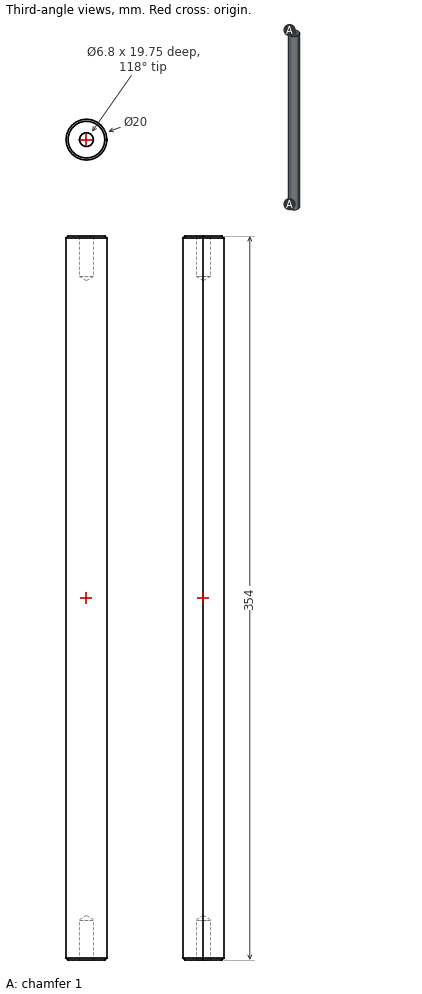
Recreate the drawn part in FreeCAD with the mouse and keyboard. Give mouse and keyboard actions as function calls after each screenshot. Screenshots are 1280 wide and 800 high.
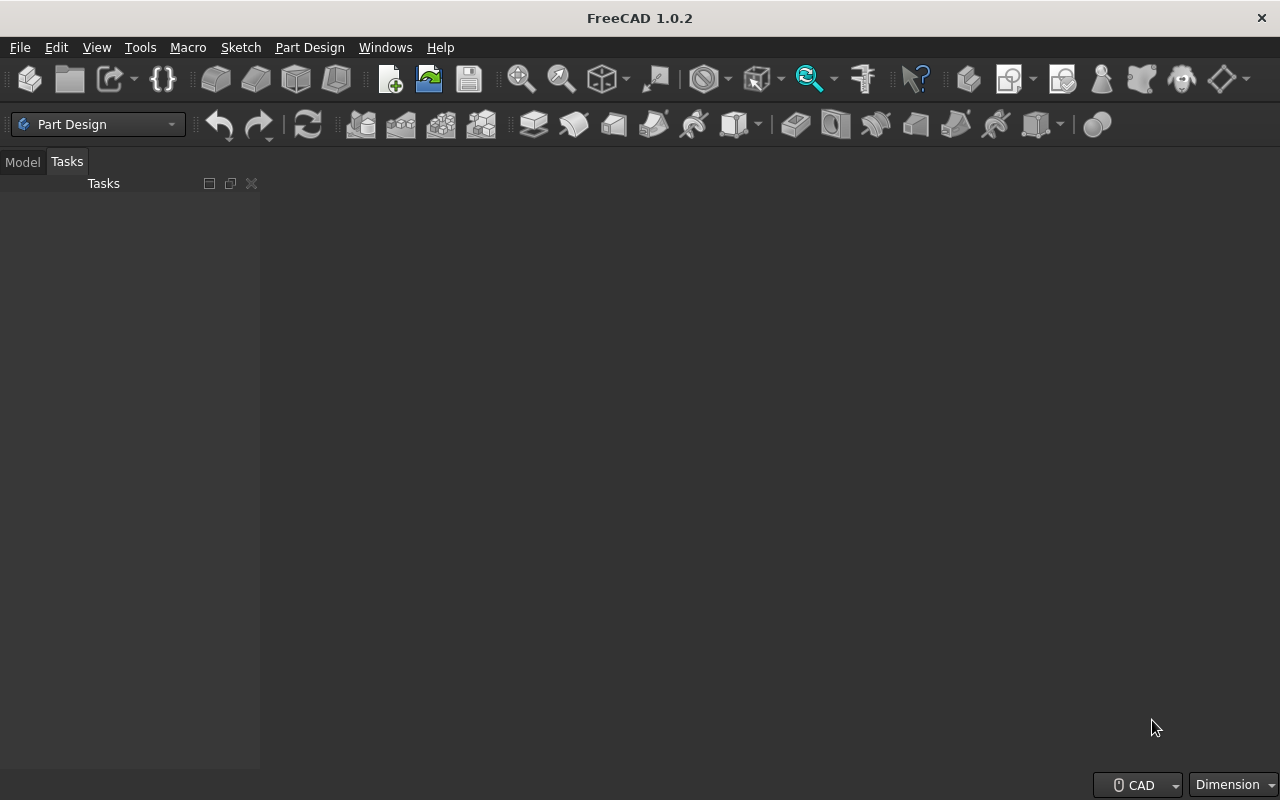
click(390, 80)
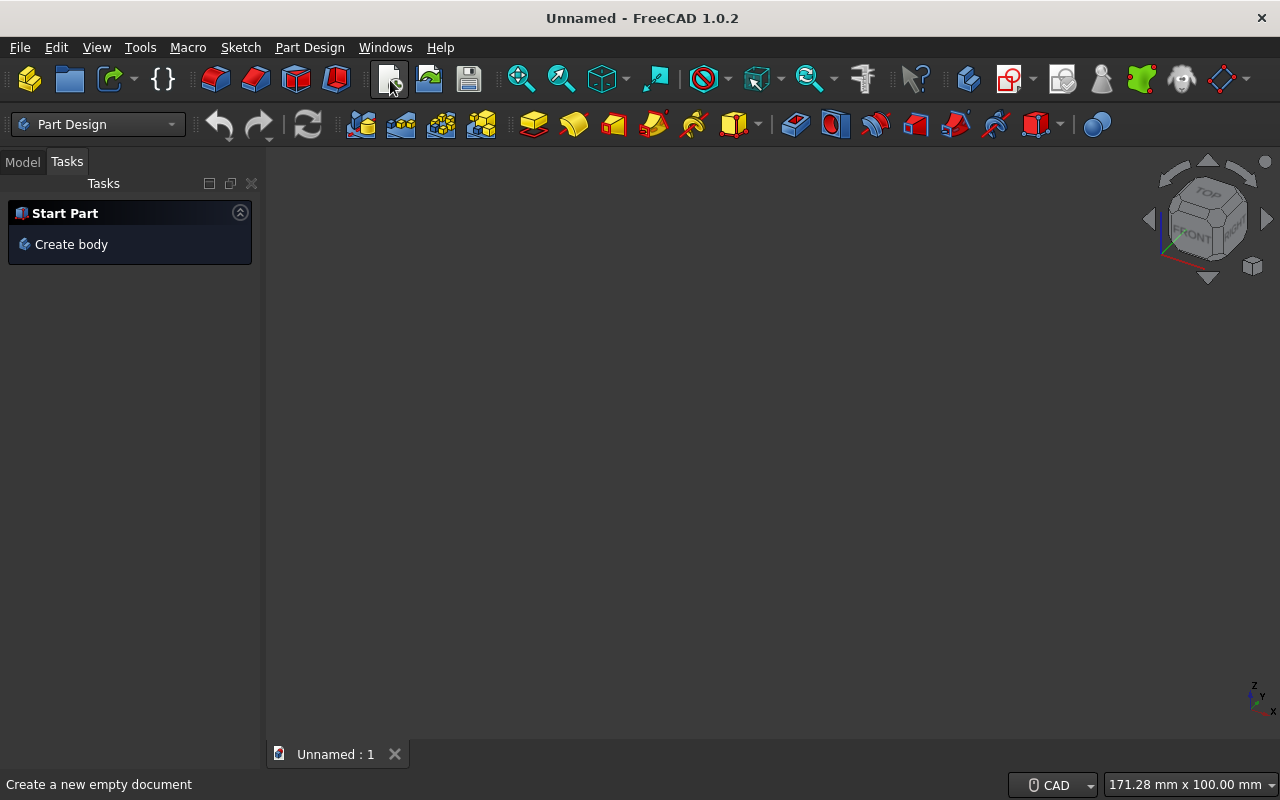
click(1010, 80)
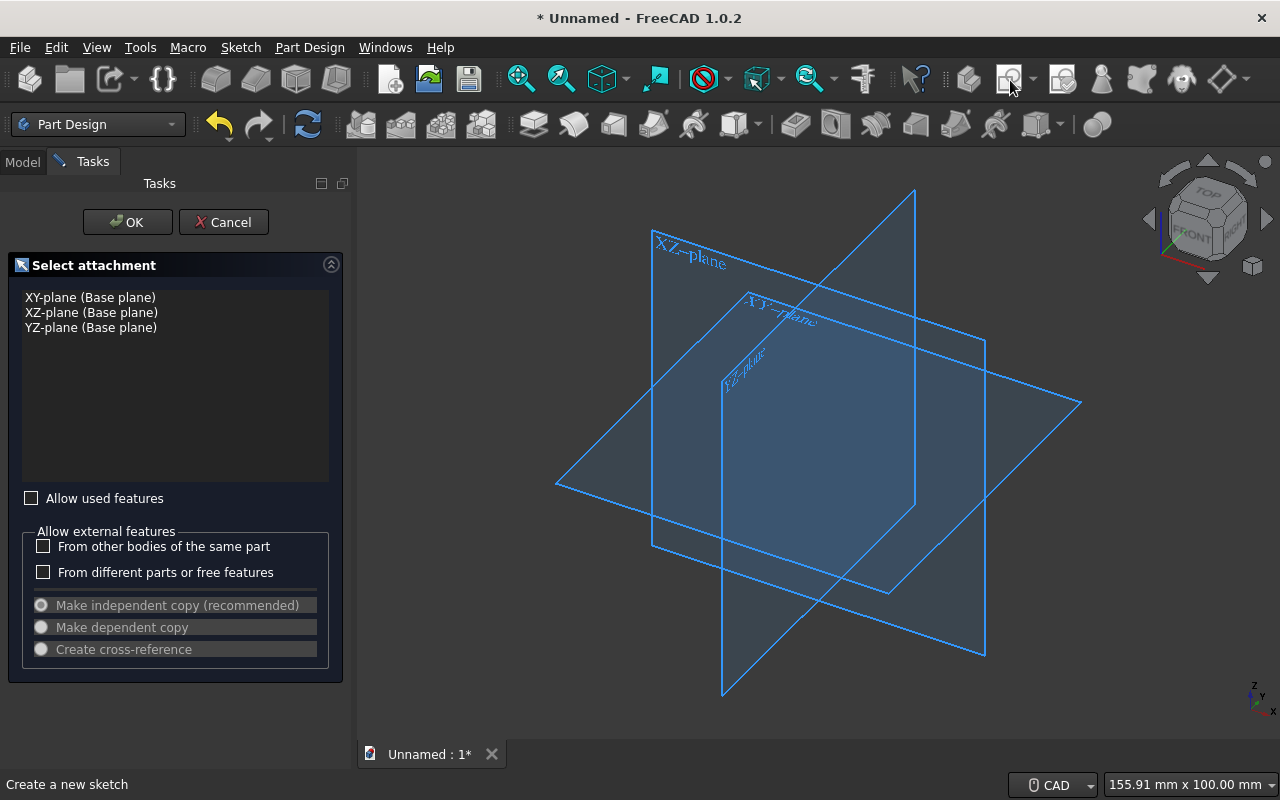
click(82, 298)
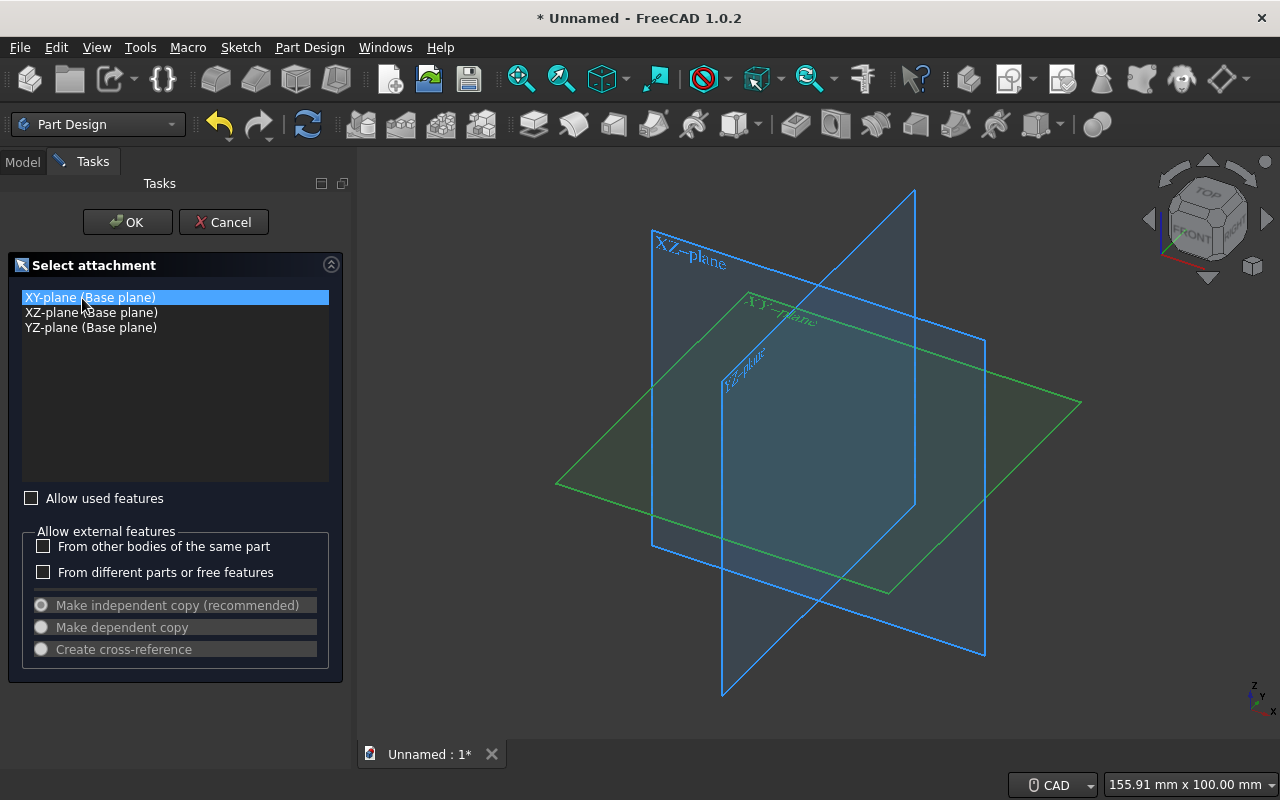
click(128, 222)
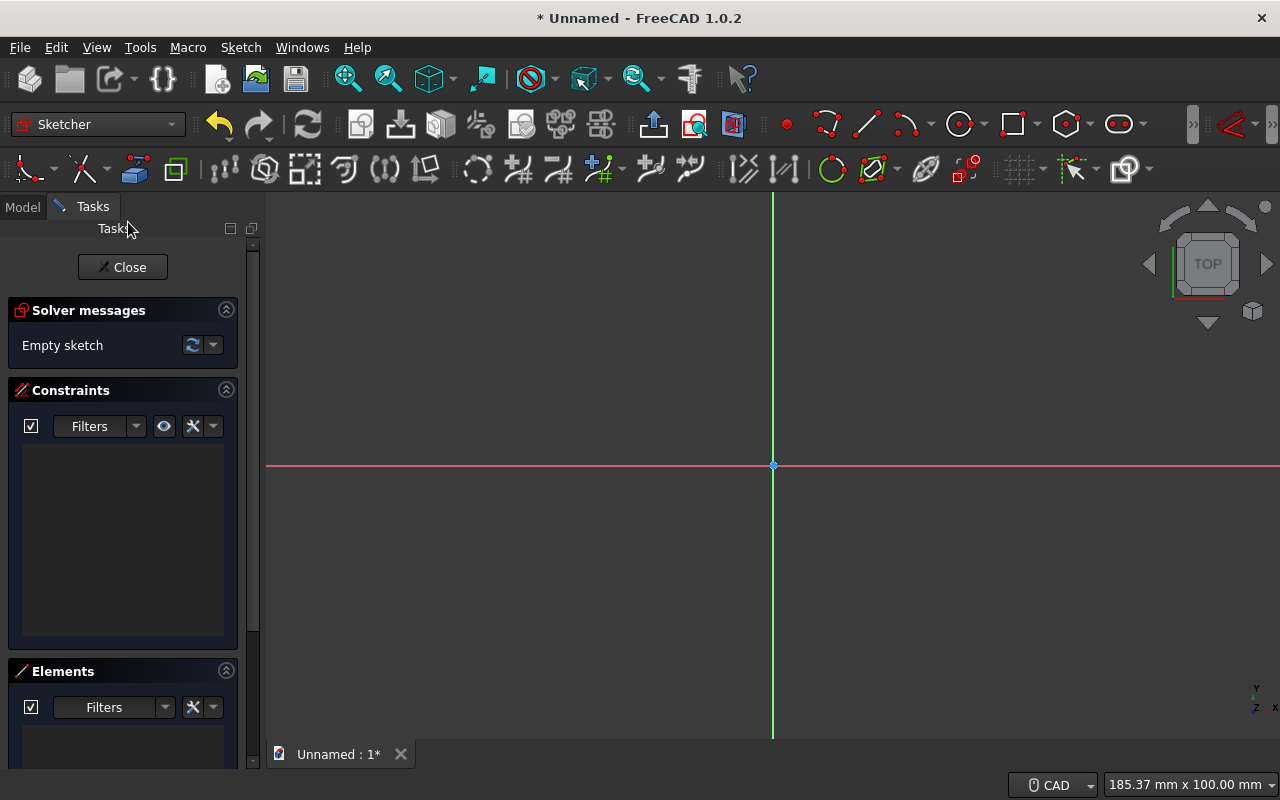
scroll(803, 466, up, 6)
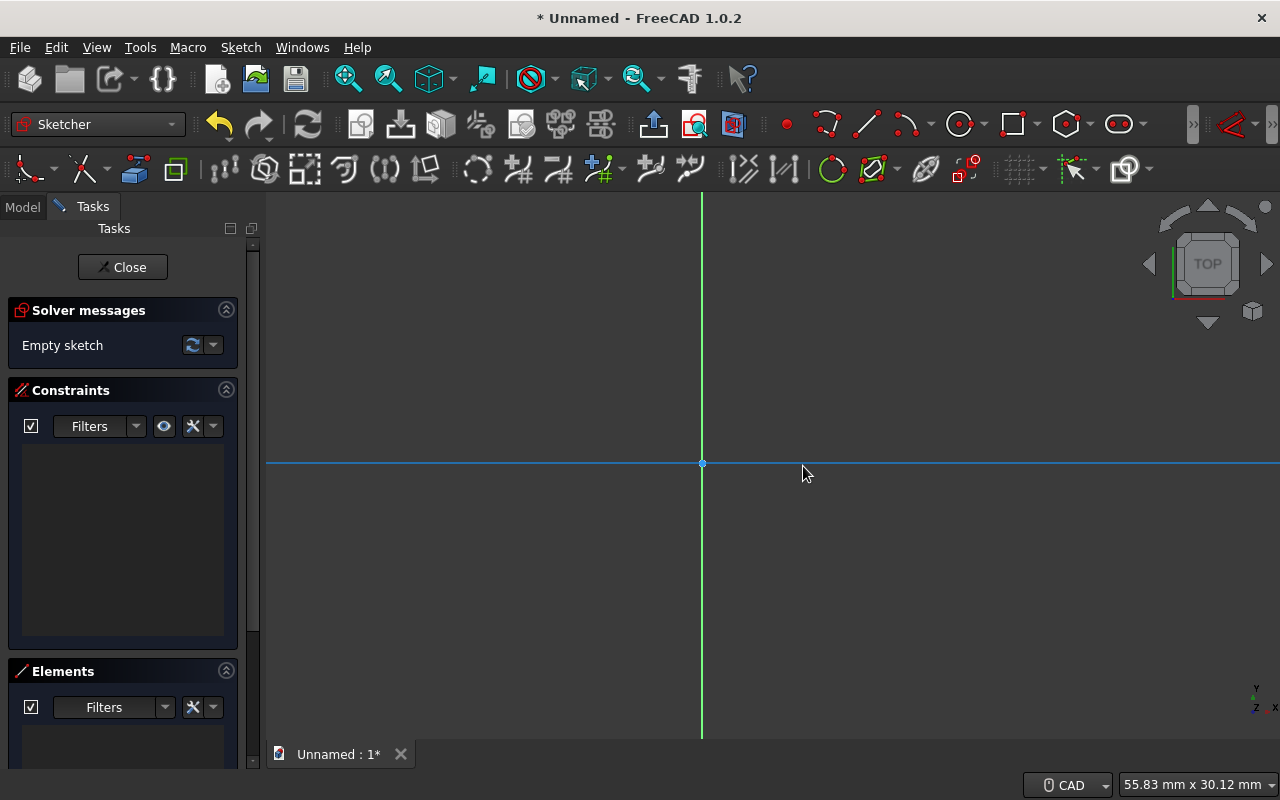
key(g)
key(c)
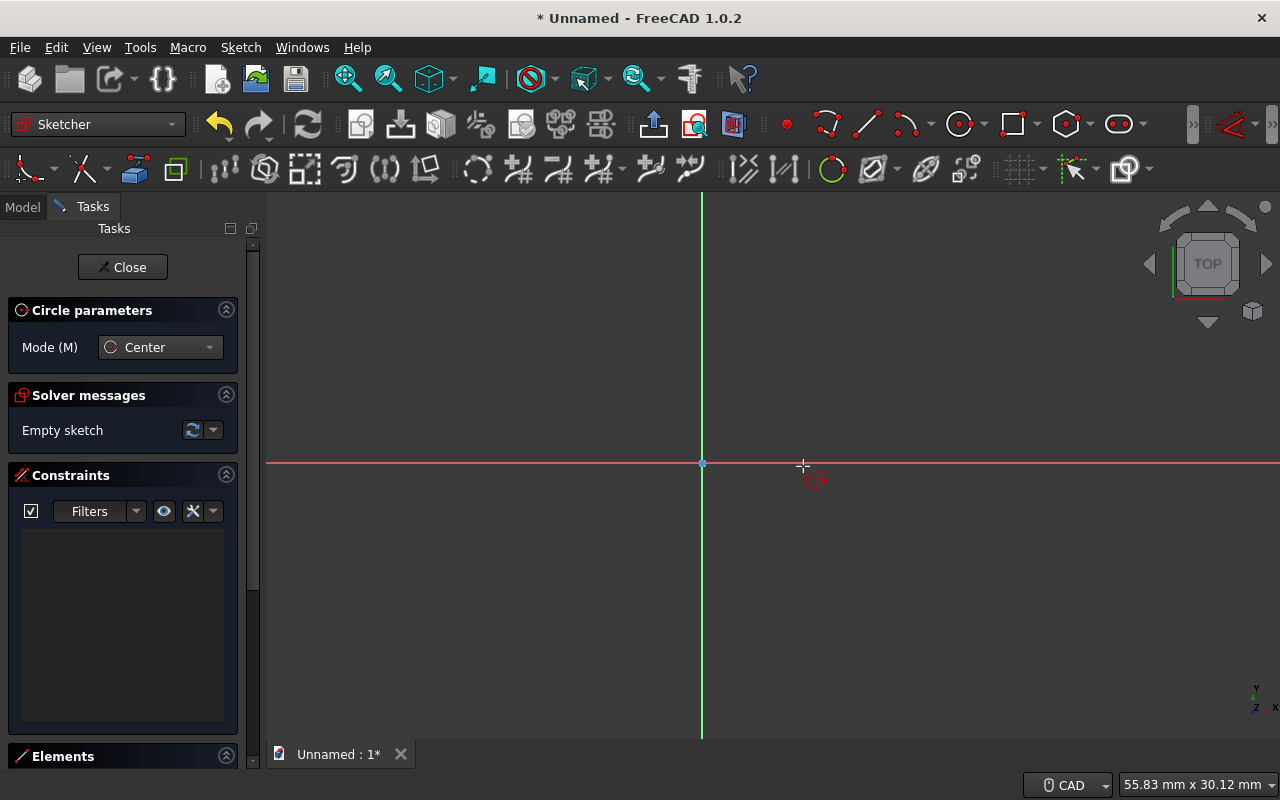
click(702, 463)
move(831, 335)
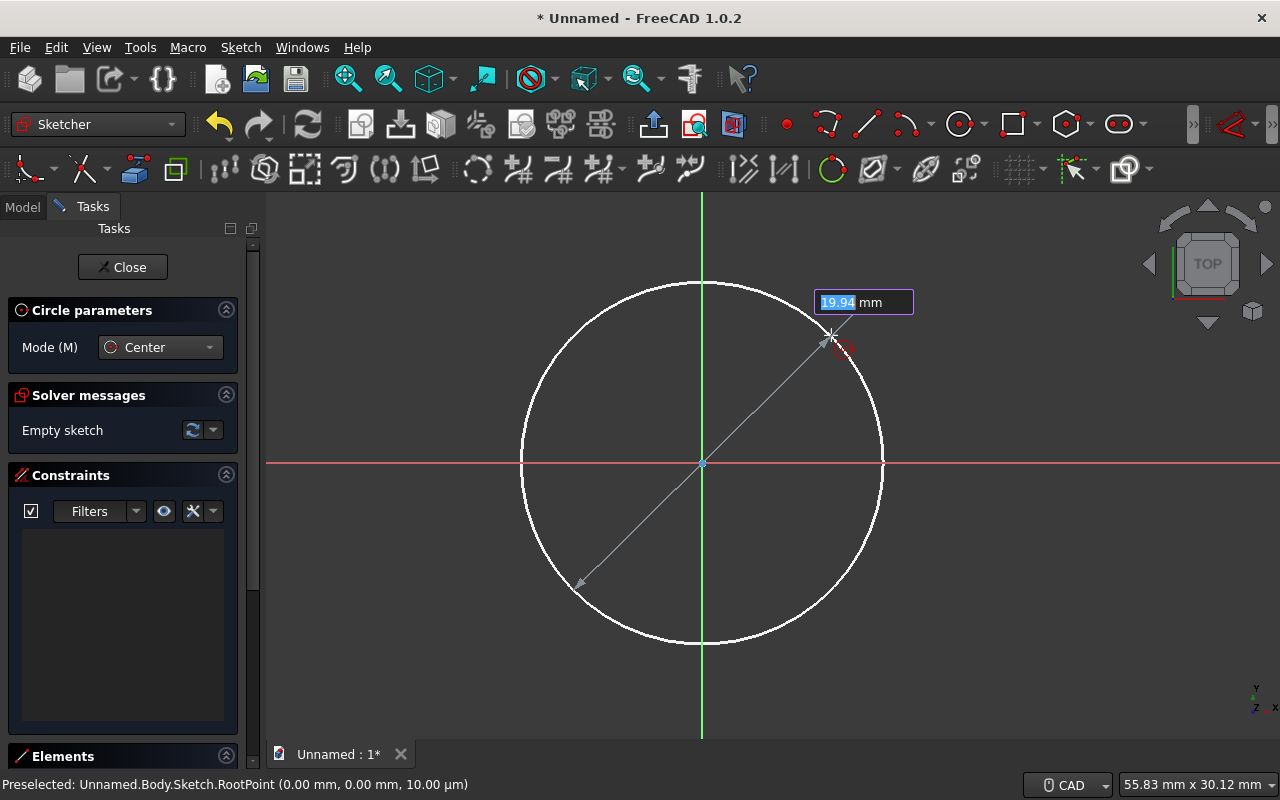
text(20)
key(Return)
key(Escape)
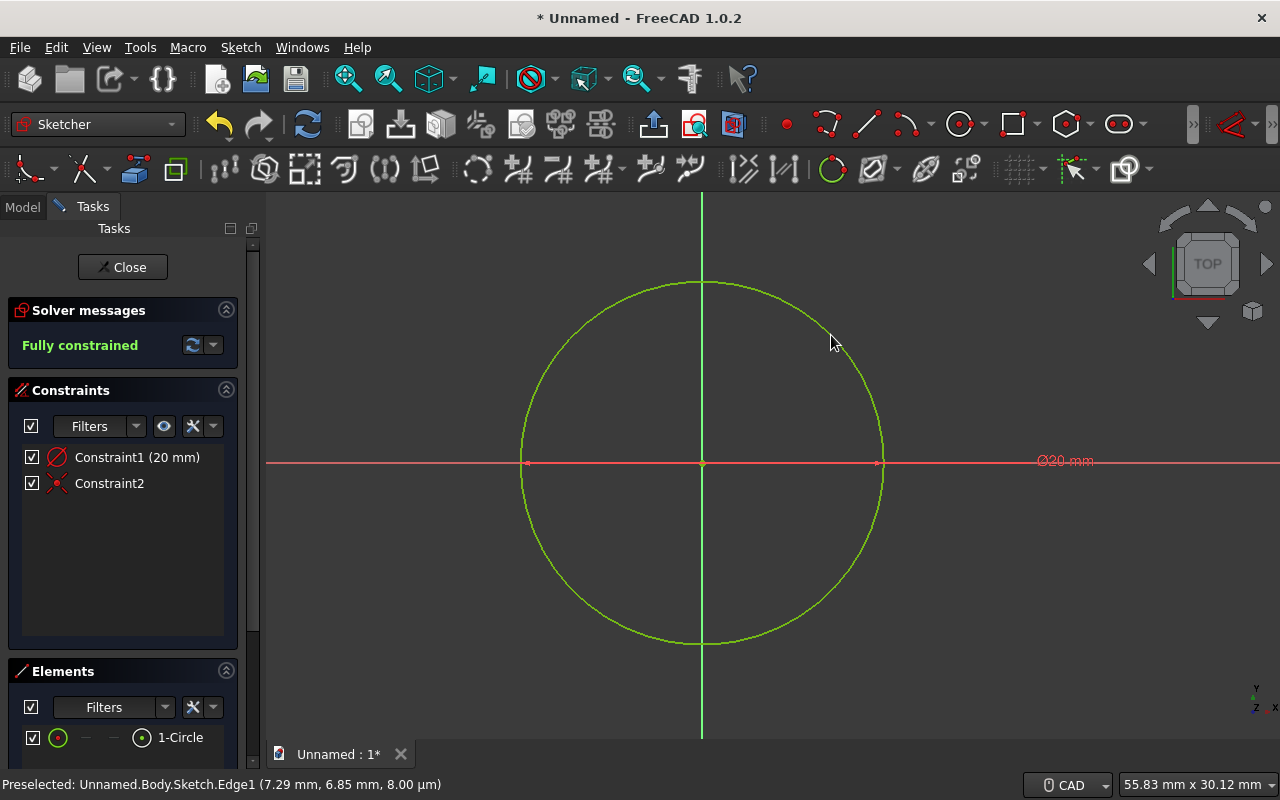
click(123, 267)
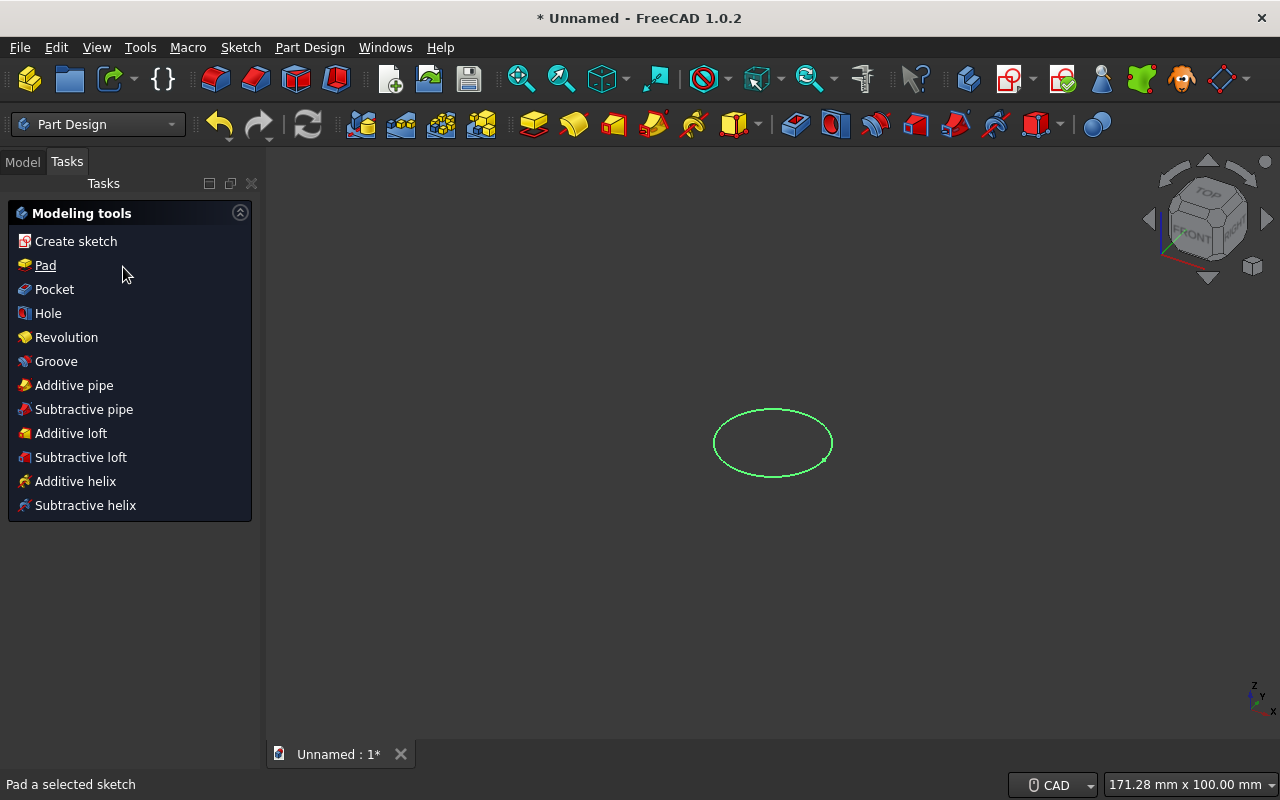
click(534, 124)